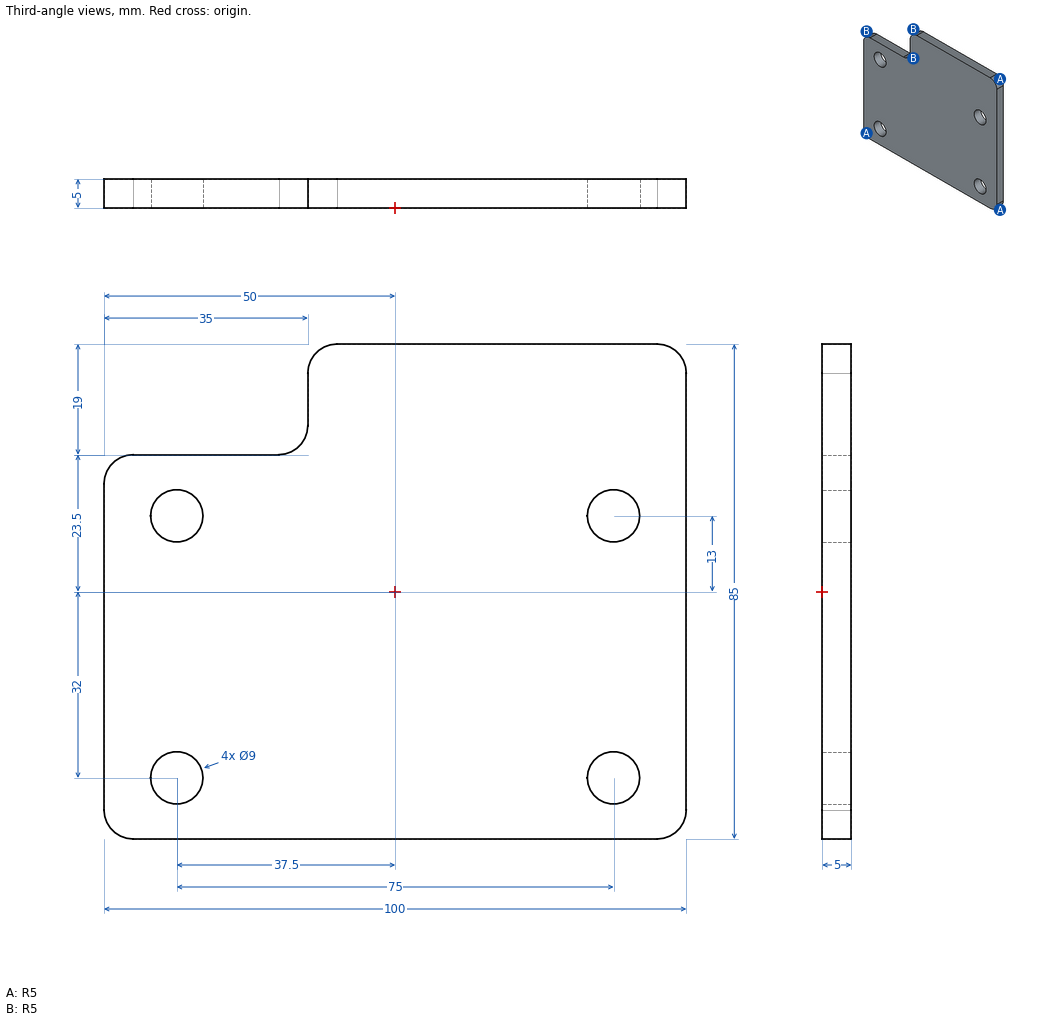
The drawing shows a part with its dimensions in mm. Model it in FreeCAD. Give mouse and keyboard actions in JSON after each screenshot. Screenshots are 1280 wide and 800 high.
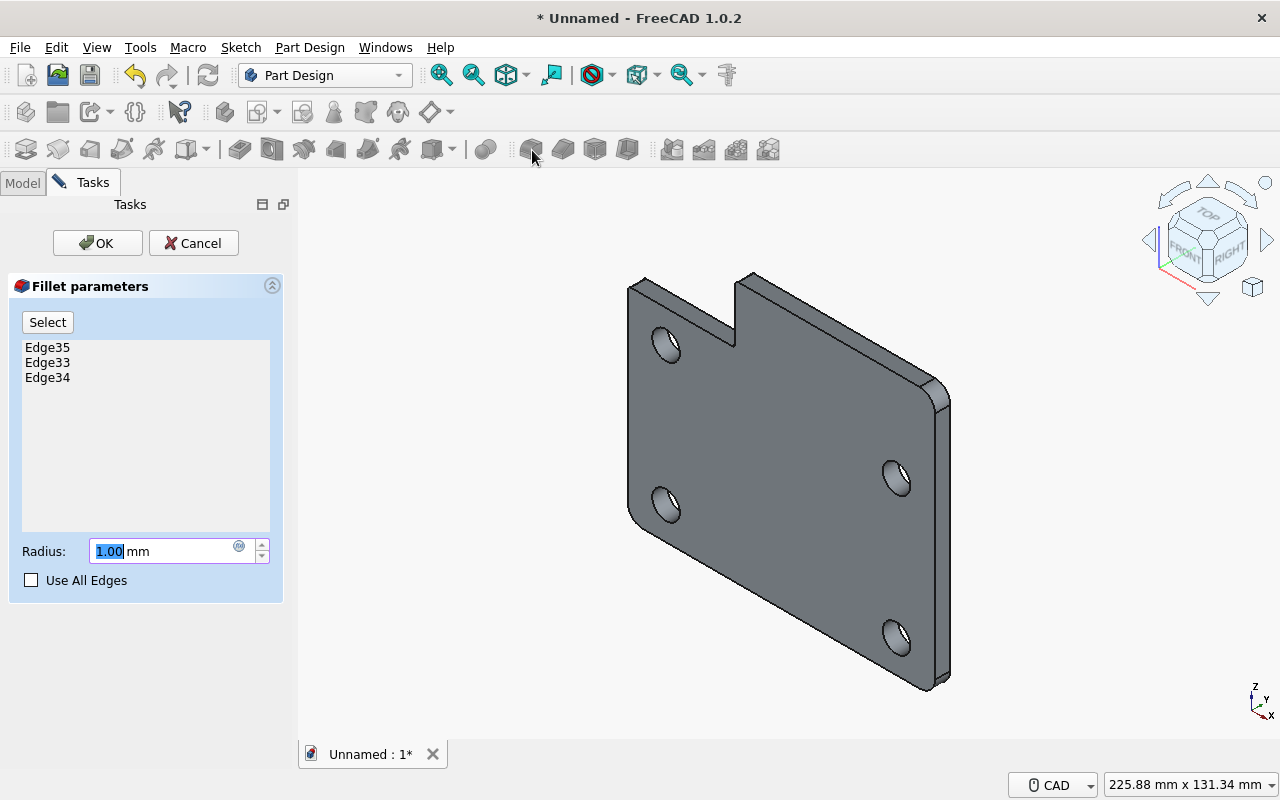
{"action": "type", "text": "5"}
{"action": "key", "text": "Tab"}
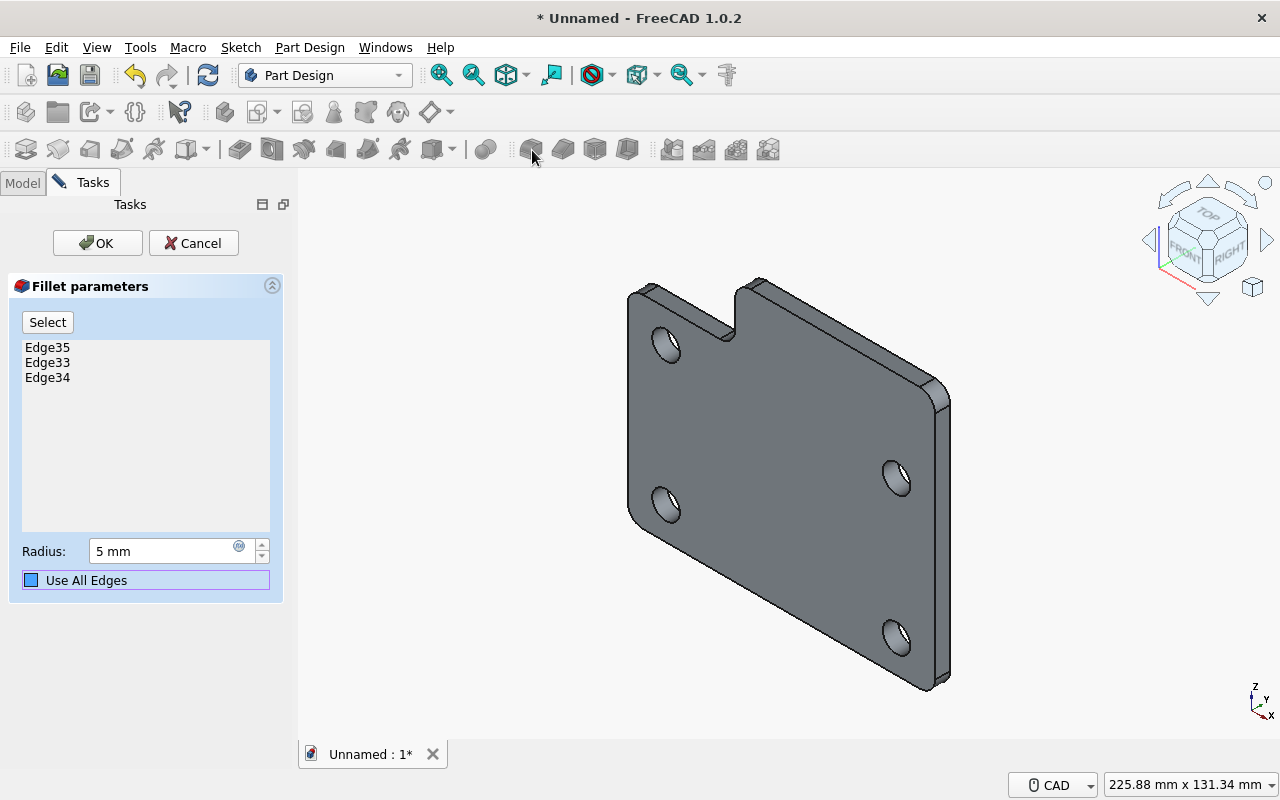
{"action": "left_click", "coordinate": [98, 243]}